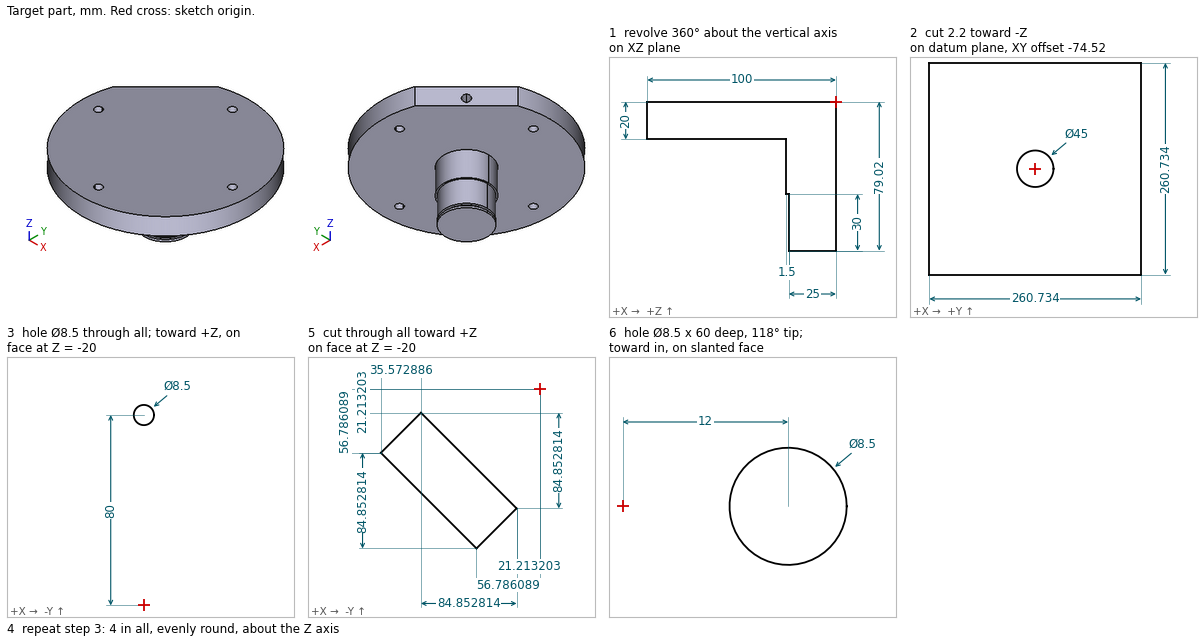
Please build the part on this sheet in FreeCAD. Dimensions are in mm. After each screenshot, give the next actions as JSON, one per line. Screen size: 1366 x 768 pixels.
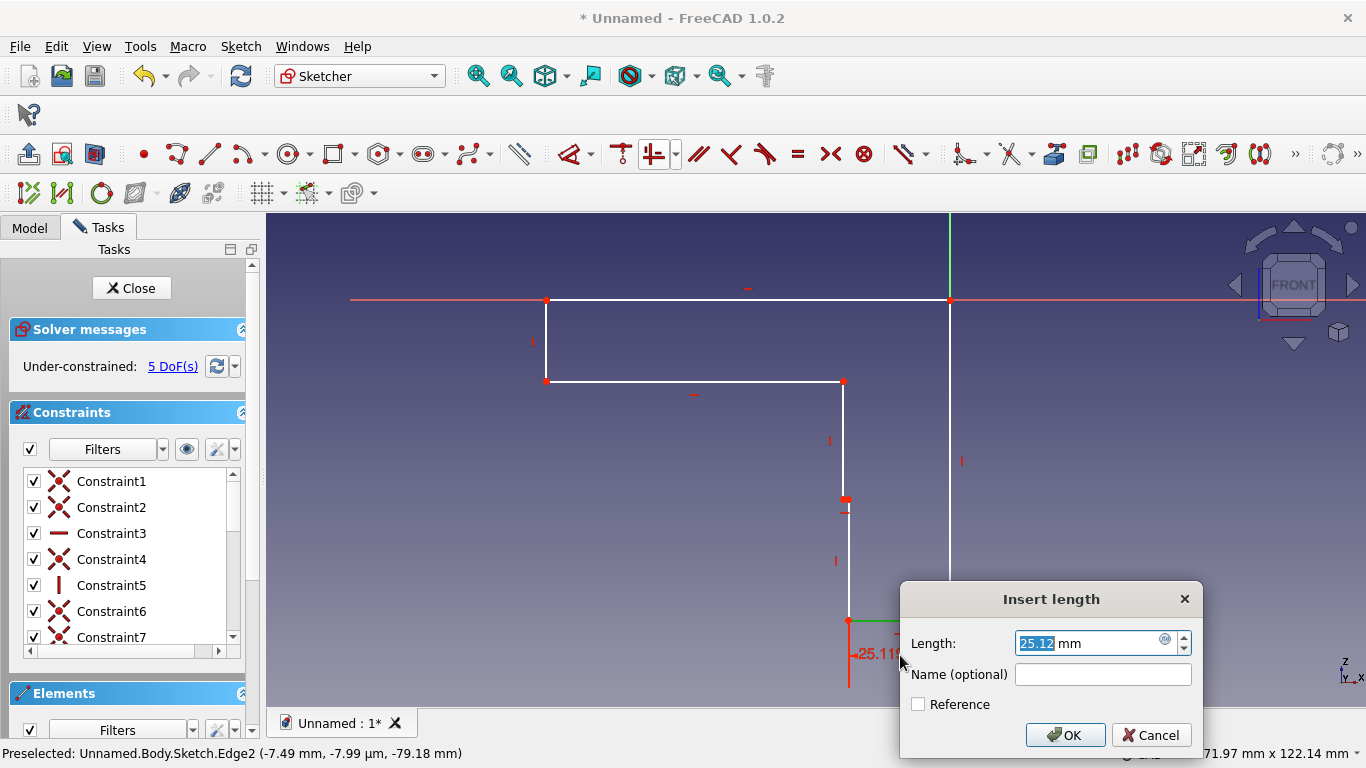
{"action": "type", "text": "25"}
{"action": "key", "text": "Return"}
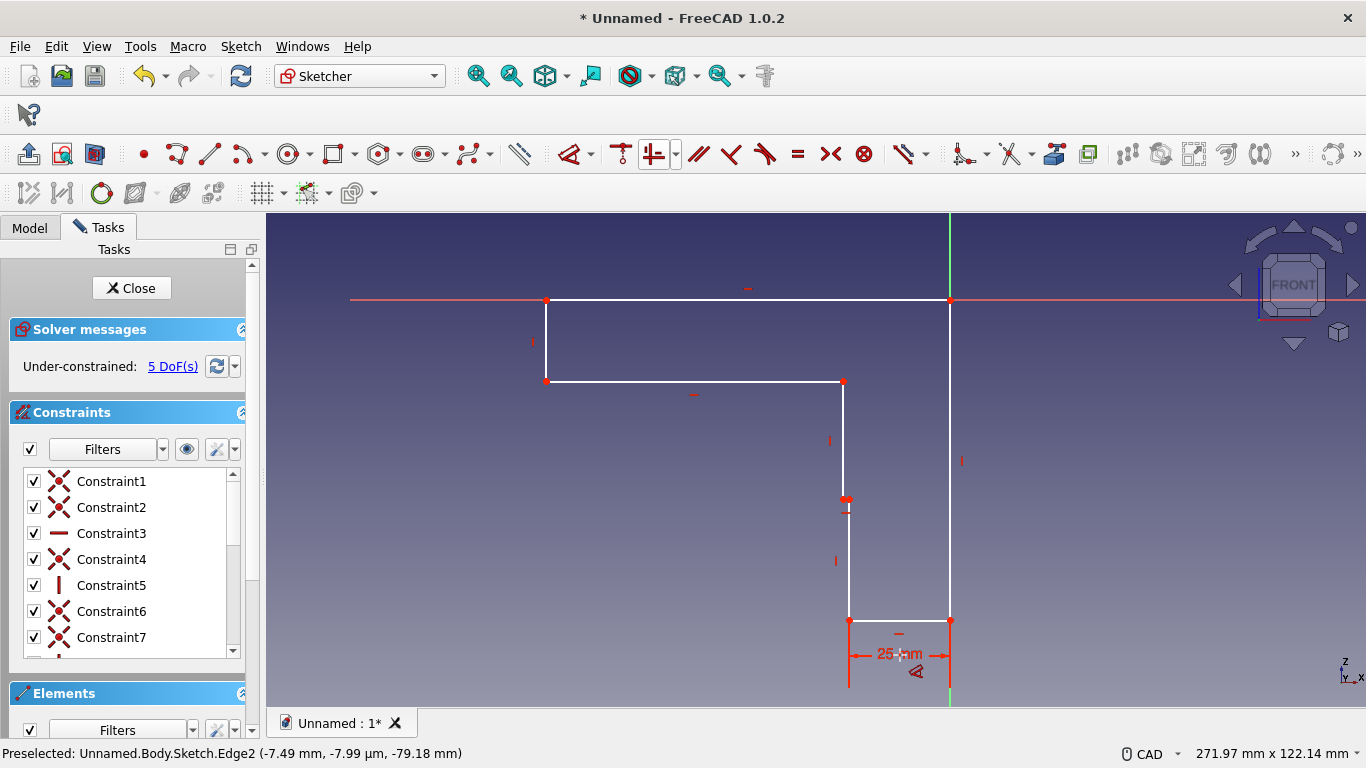
{"action": "left_click", "coordinate": [849, 584]}
{"action": "left_click", "coordinate": [883, 560]}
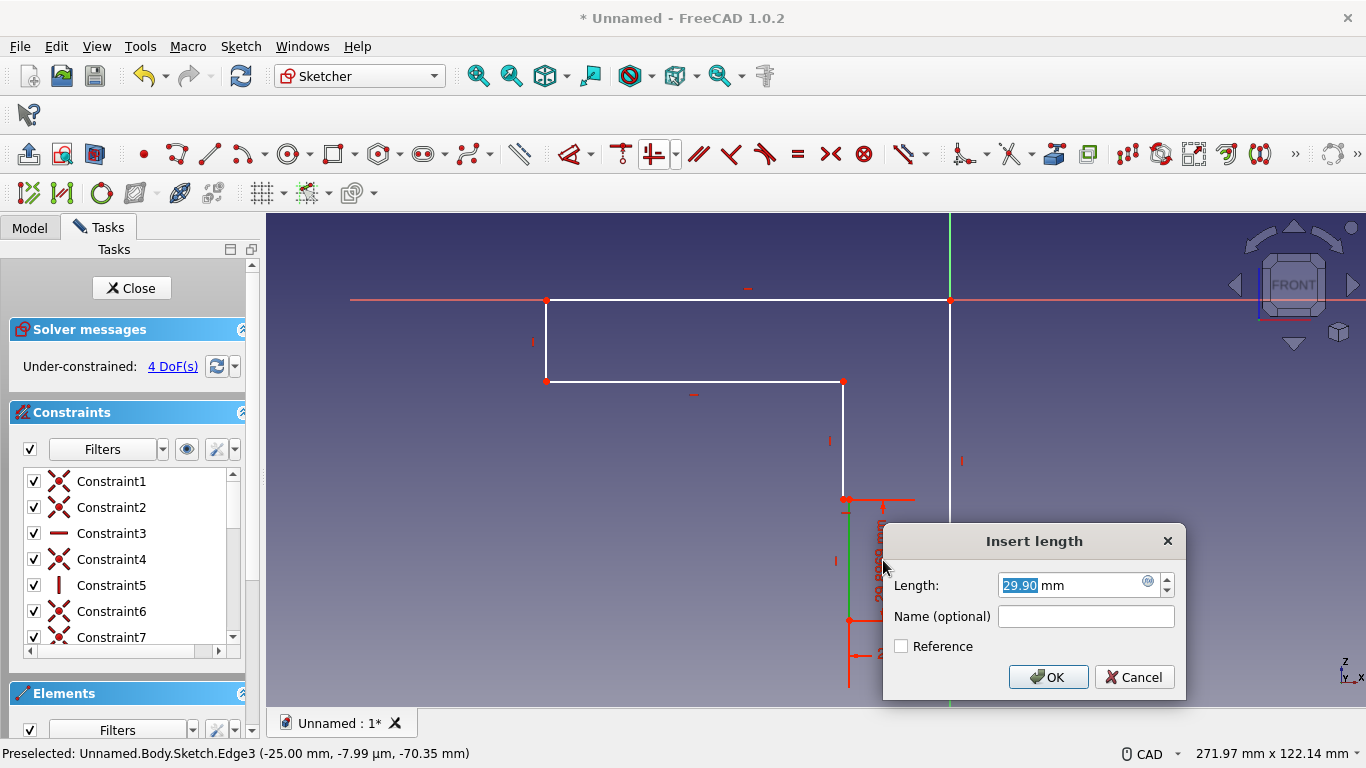
{"action": "type", "text": "30"}
{"action": "key", "text": "Return"}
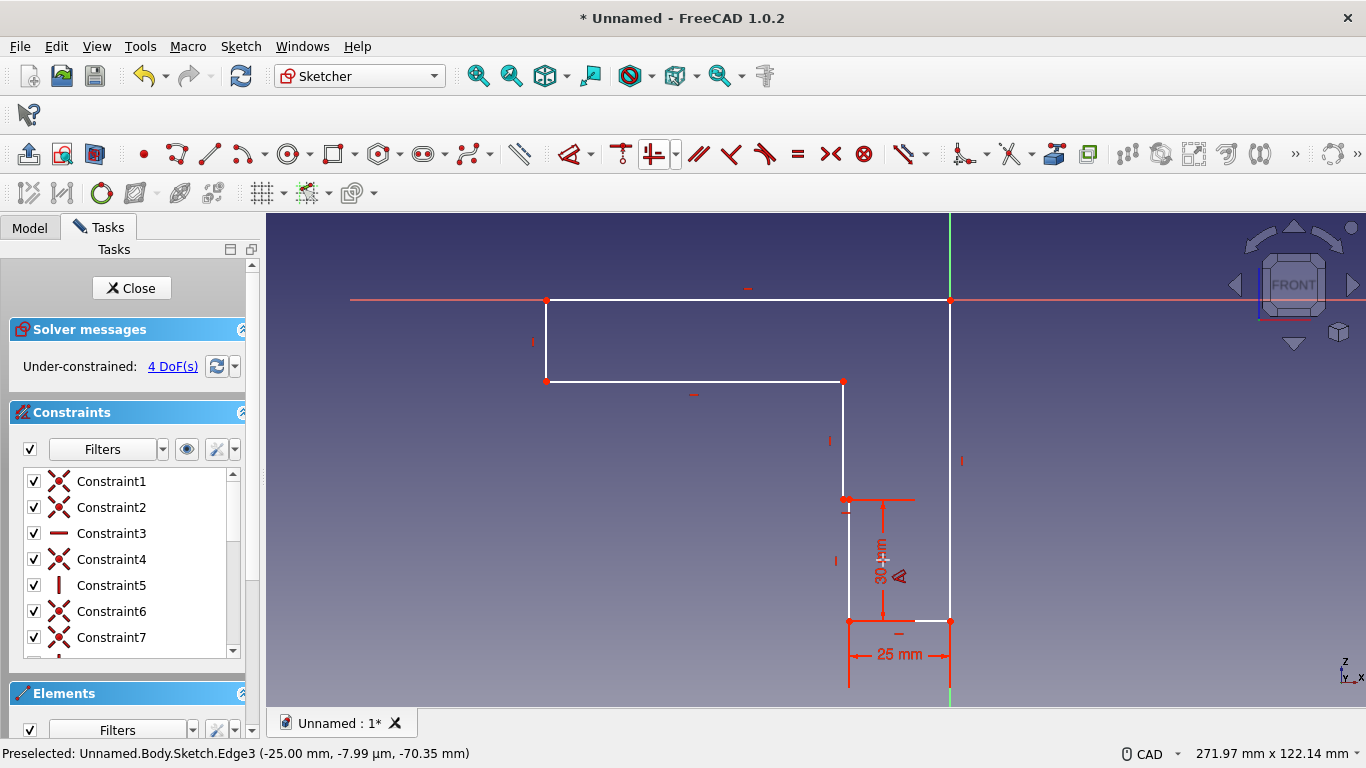
{"action": "left_click", "coordinate": [546, 358]}
{"action": "left_click", "coordinate": [512, 341]}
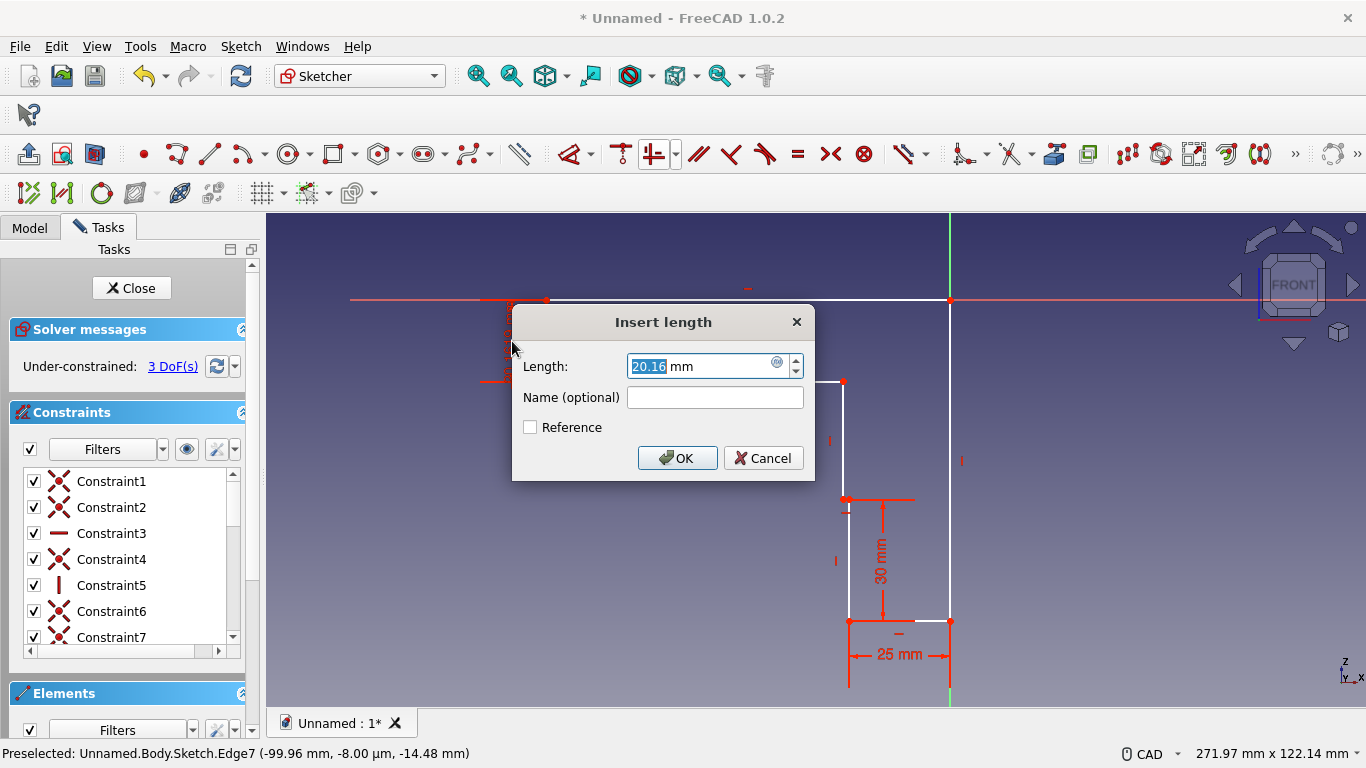
{"action": "type", "text": "20"}
{"action": "key", "text": "Return"}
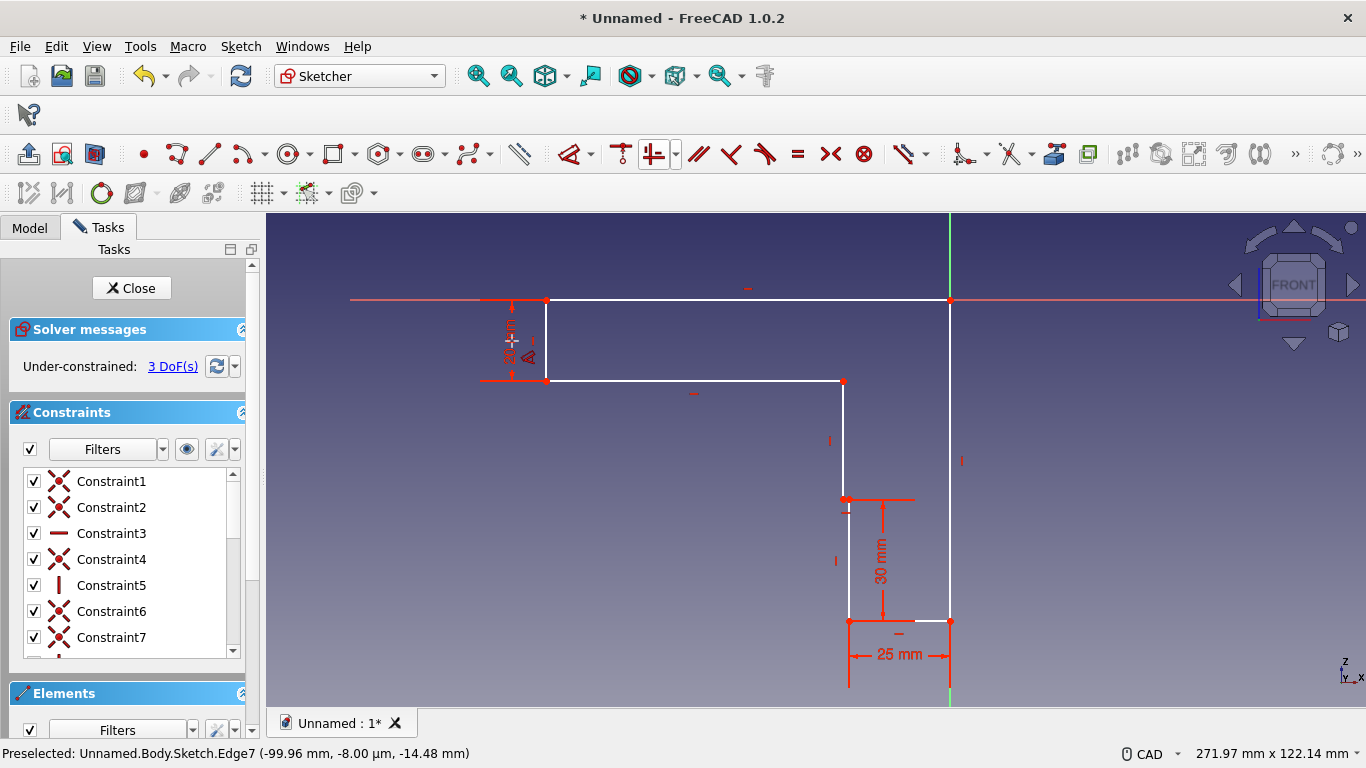
{"action": "scroll", "coordinate": [846, 500], "scroll_direction": "up", "scroll_amount": 10}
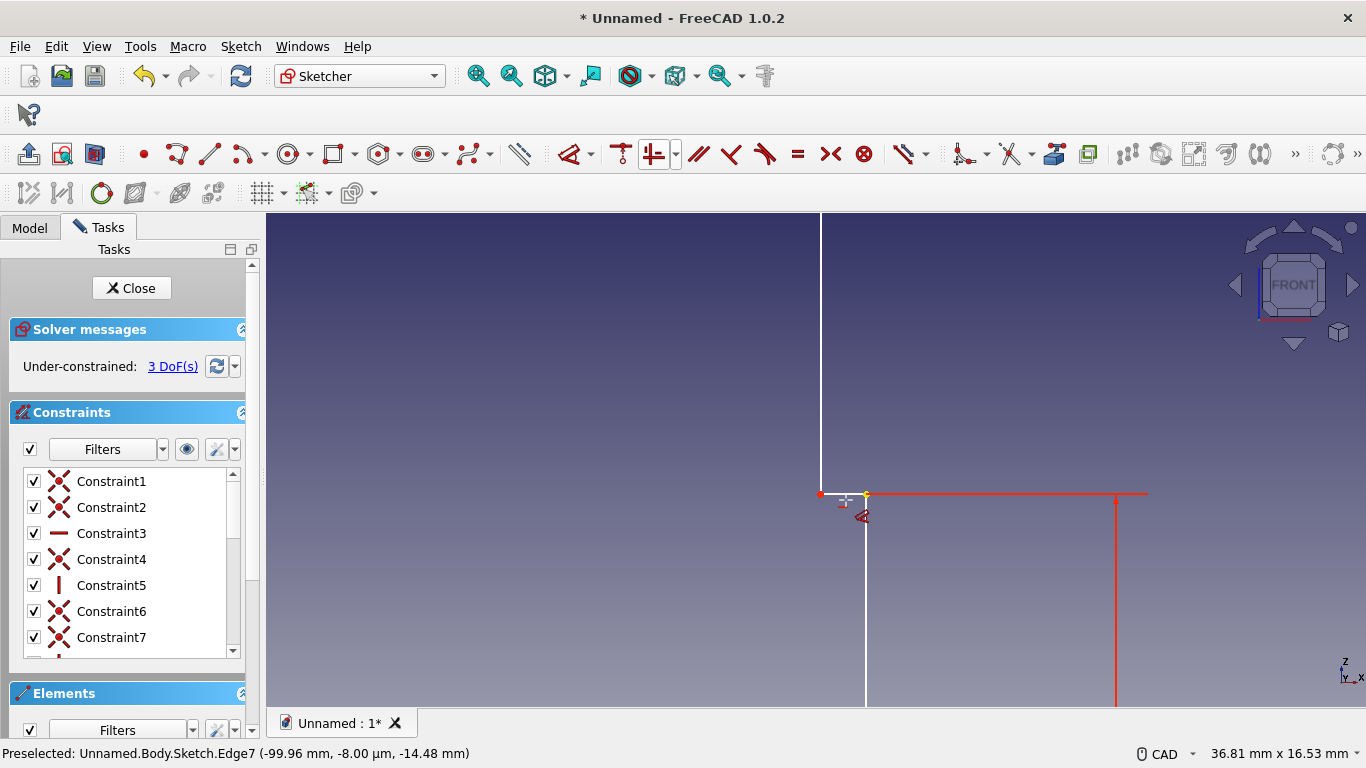
{"action": "left_click", "coordinate": [843, 494]}
{"action": "left_click", "coordinate": [843, 528]}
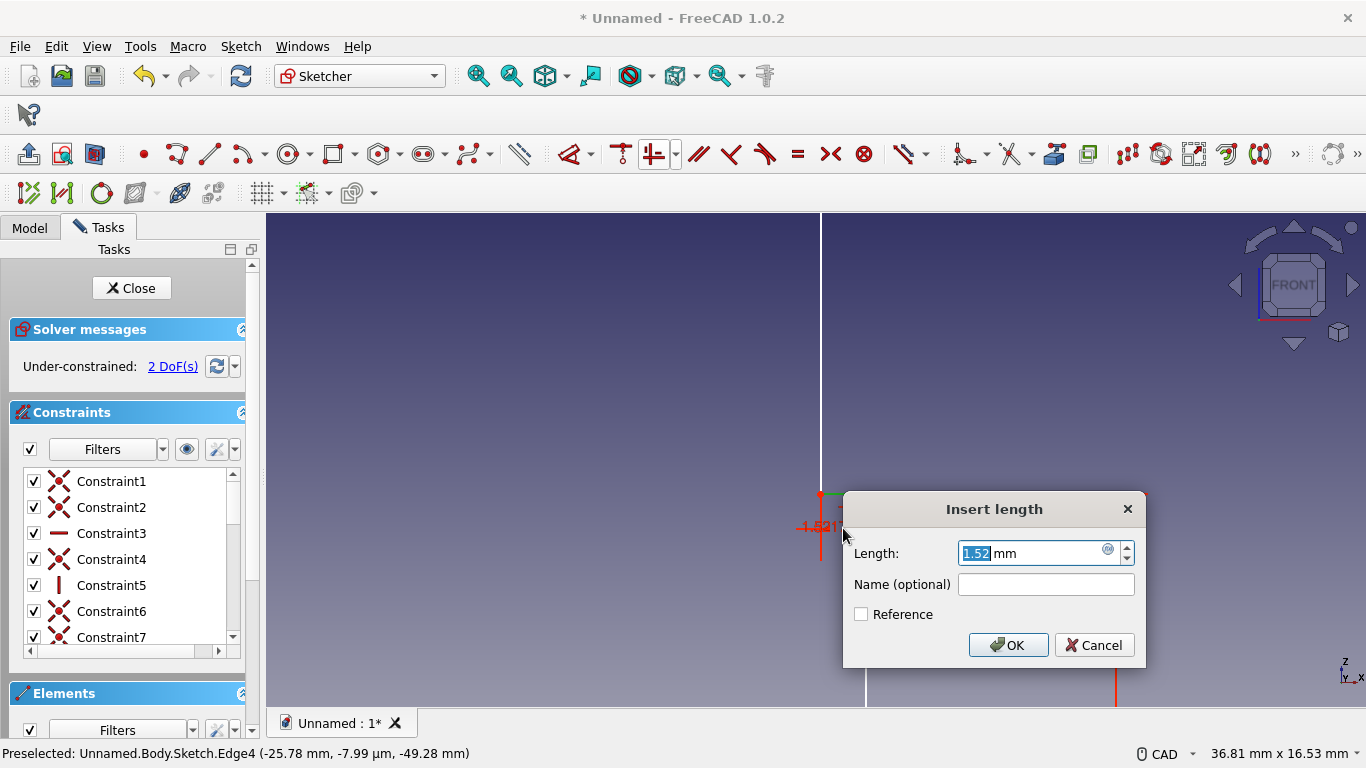
{"action": "type", "text": "1.5"}
{"action": "key", "text": "Return"}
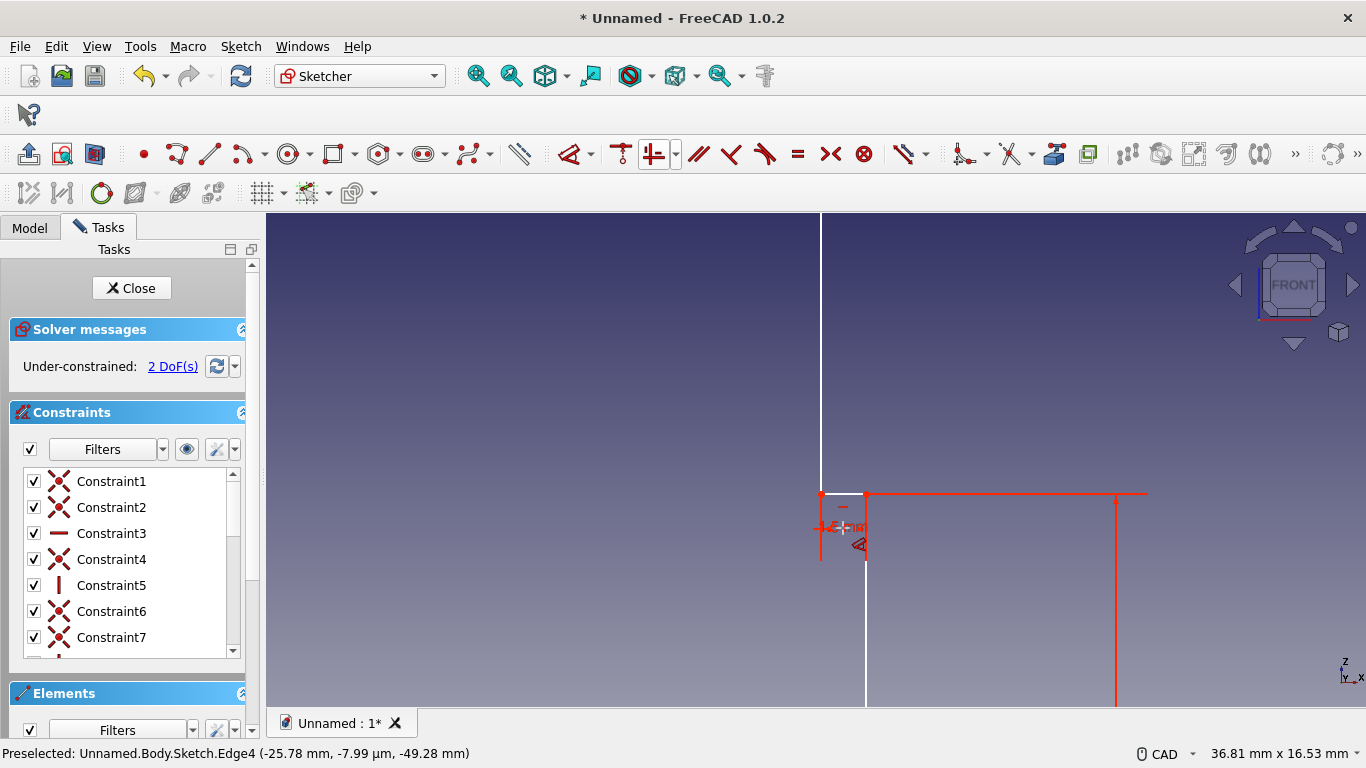
{"action": "scroll", "coordinate": [846, 500], "scroll_direction": "down", "scroll_amount": 10}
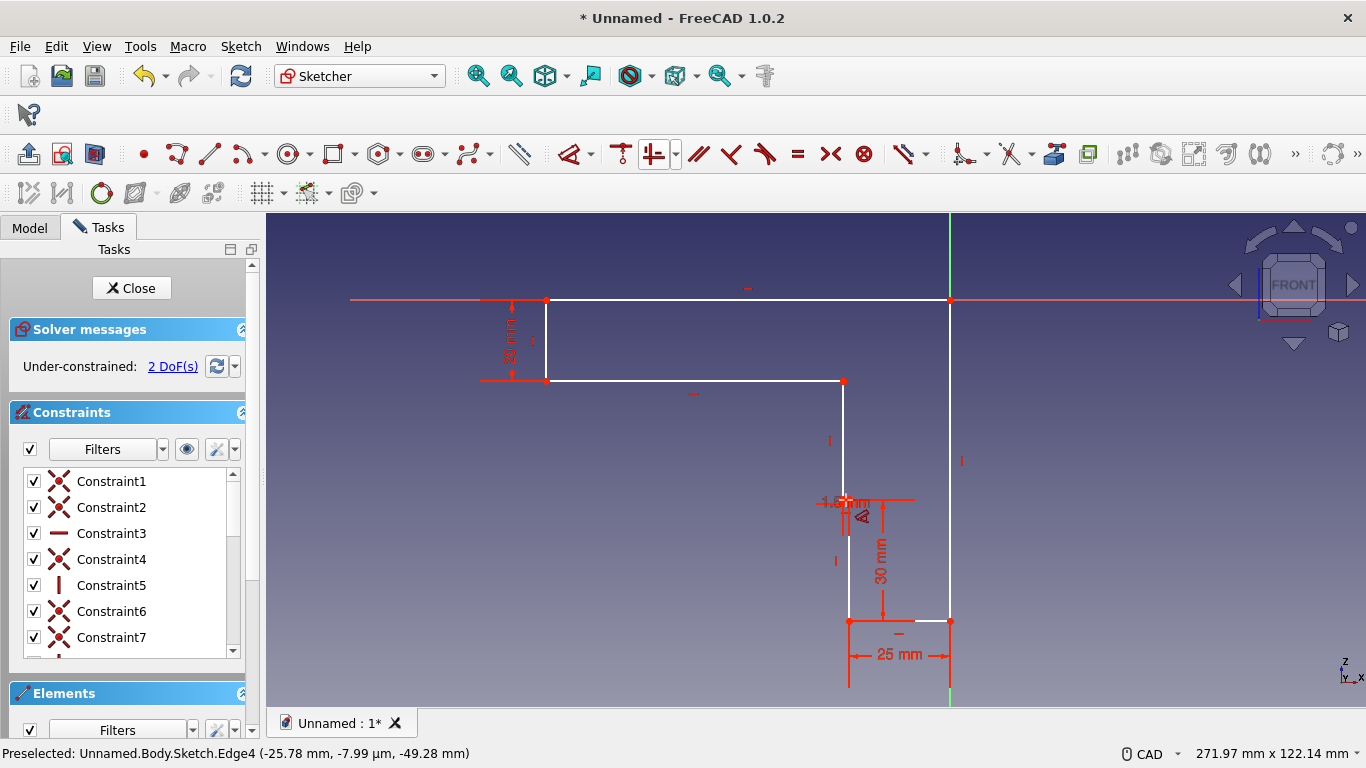
{"action": "left_click", "coordinate": [667, 300]}
{"action": "left_click", "coordinate": [748, 266]}